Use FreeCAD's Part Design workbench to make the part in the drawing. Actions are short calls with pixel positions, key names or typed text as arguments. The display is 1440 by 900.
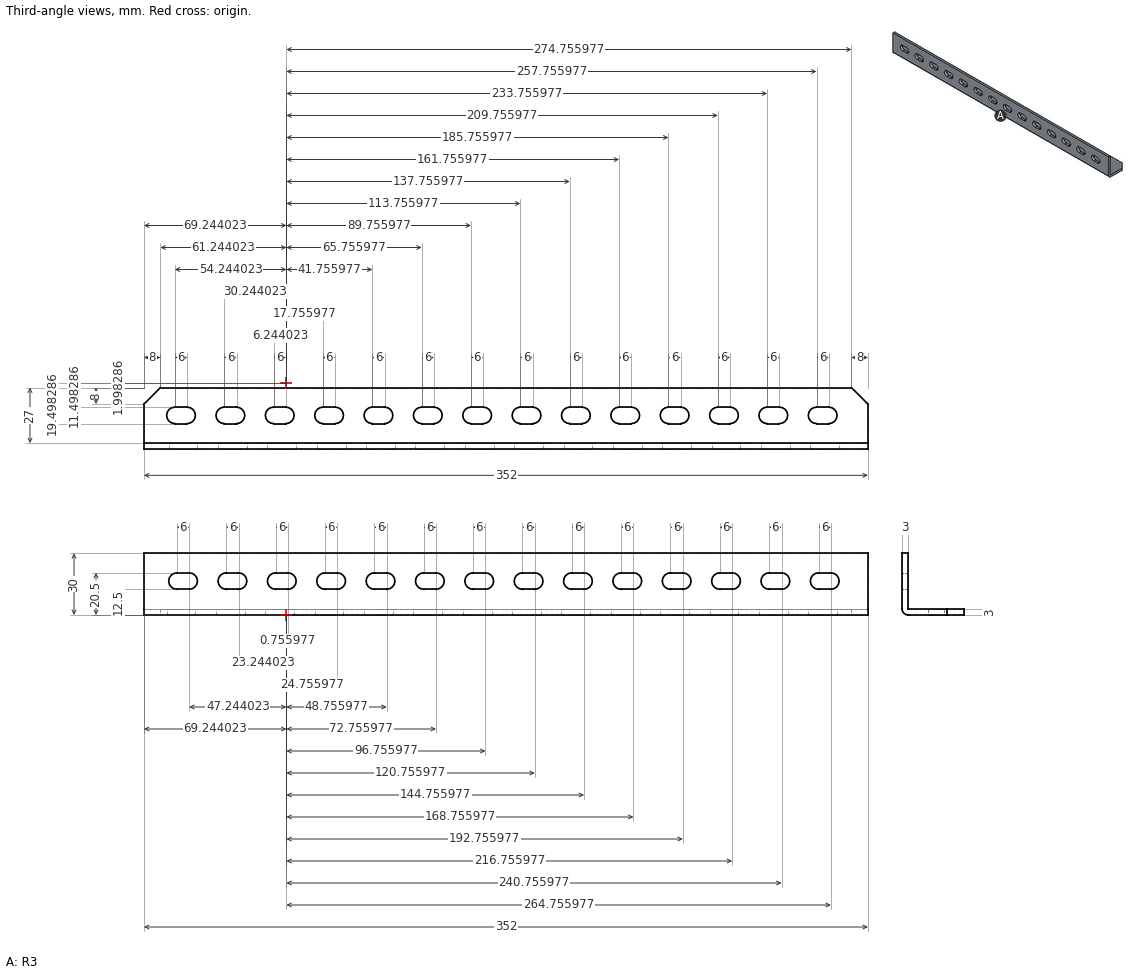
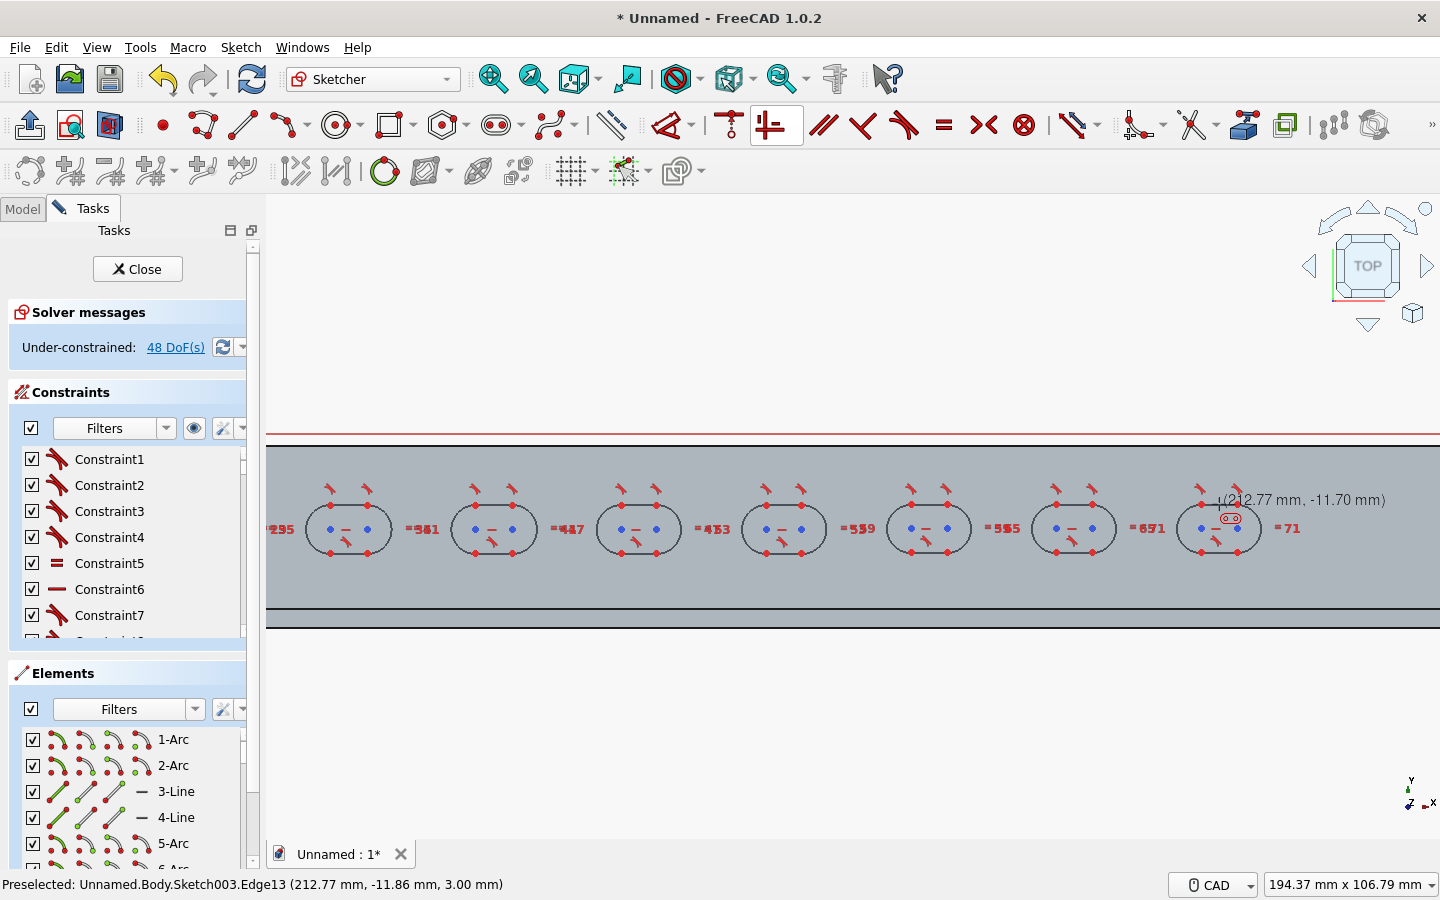
scroll(911, 530, down, 5)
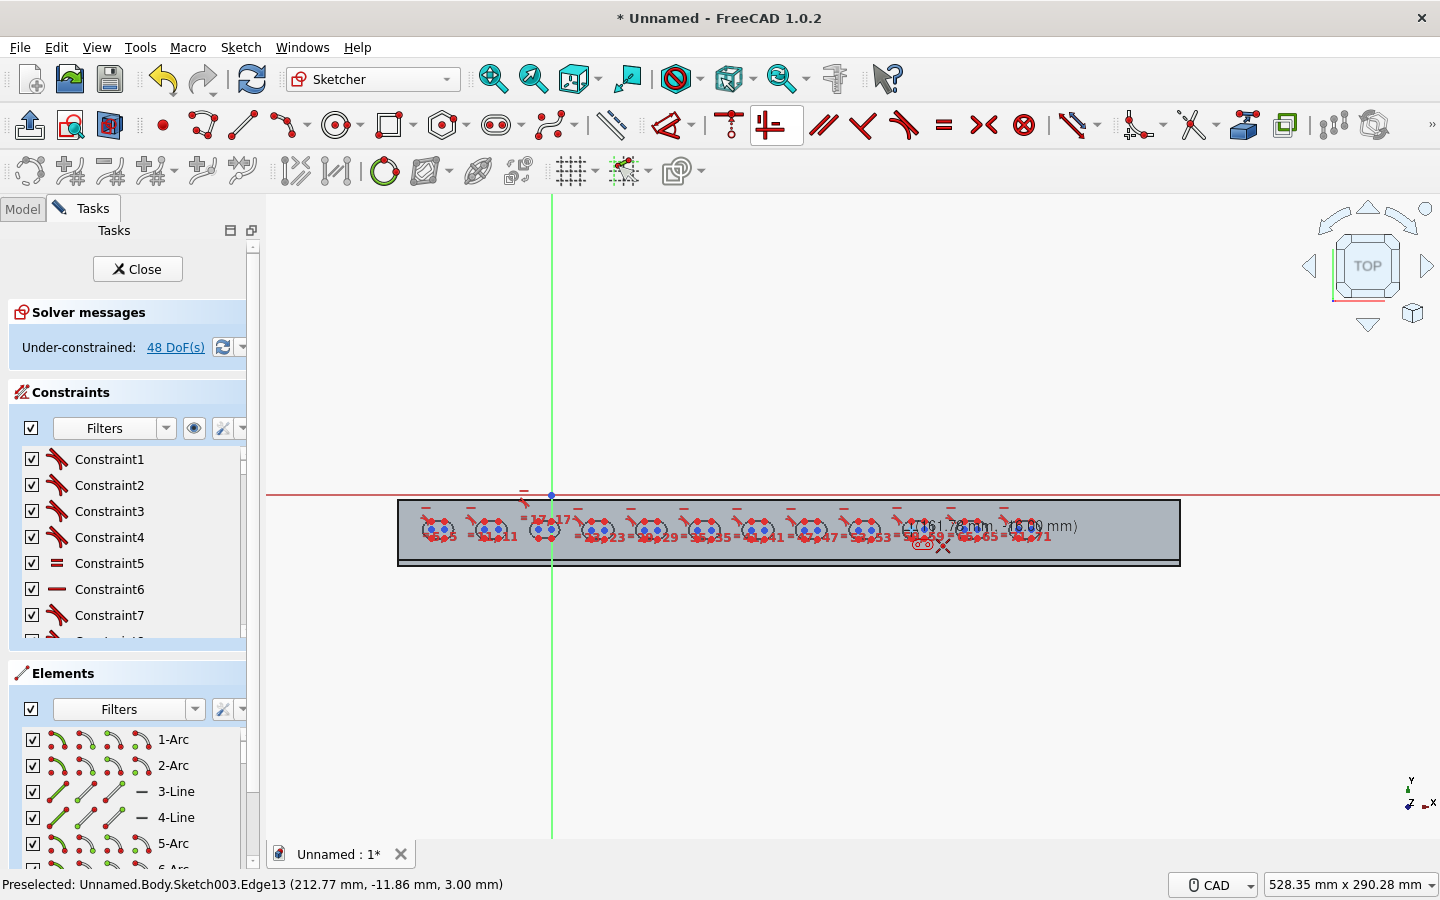
scroll(1071, 530, up, 5)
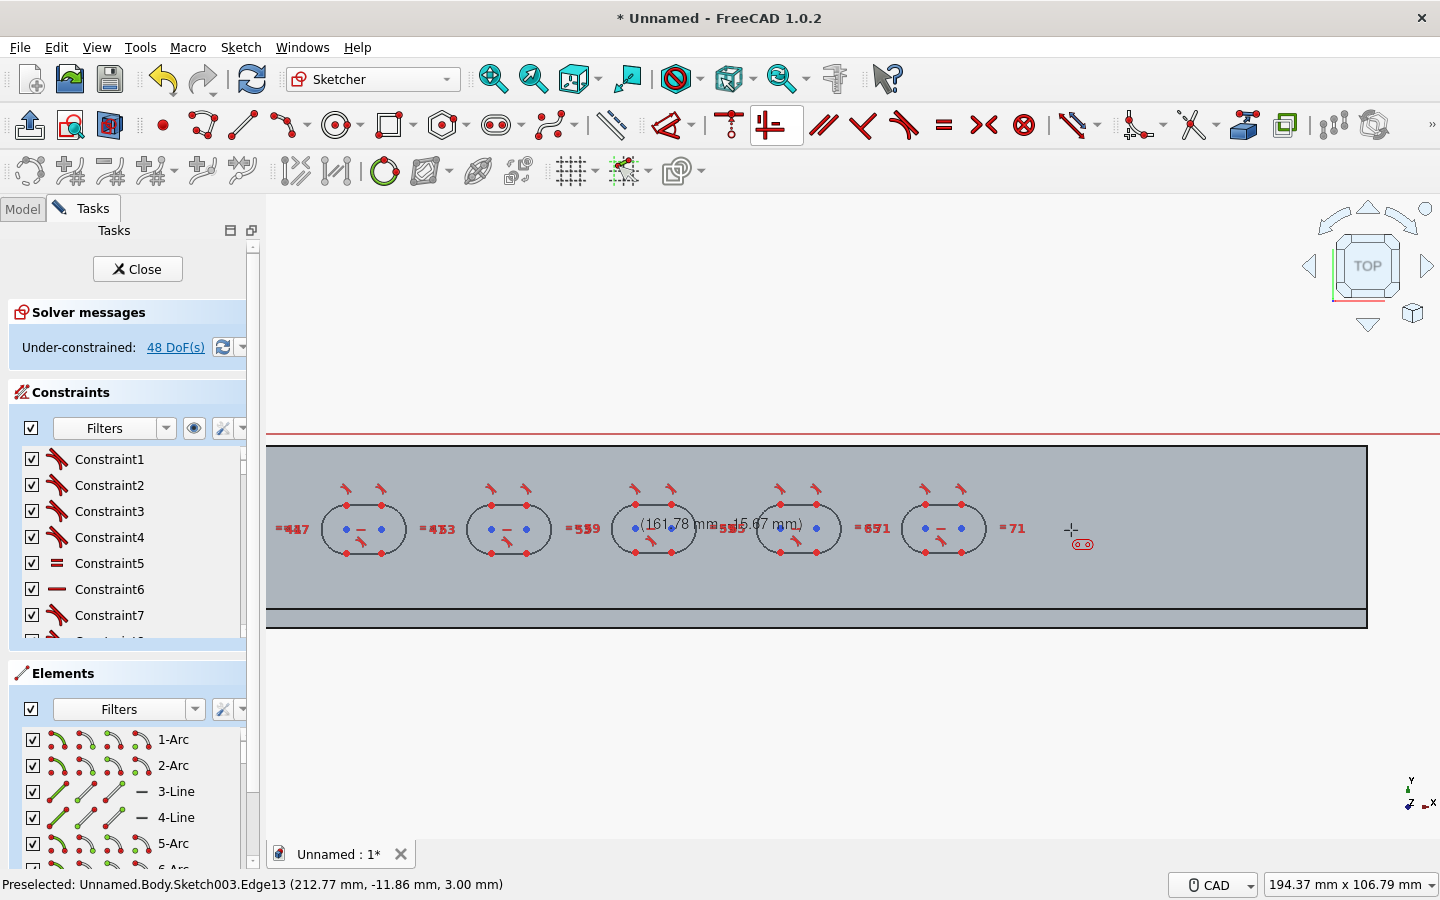
click(1071, 528)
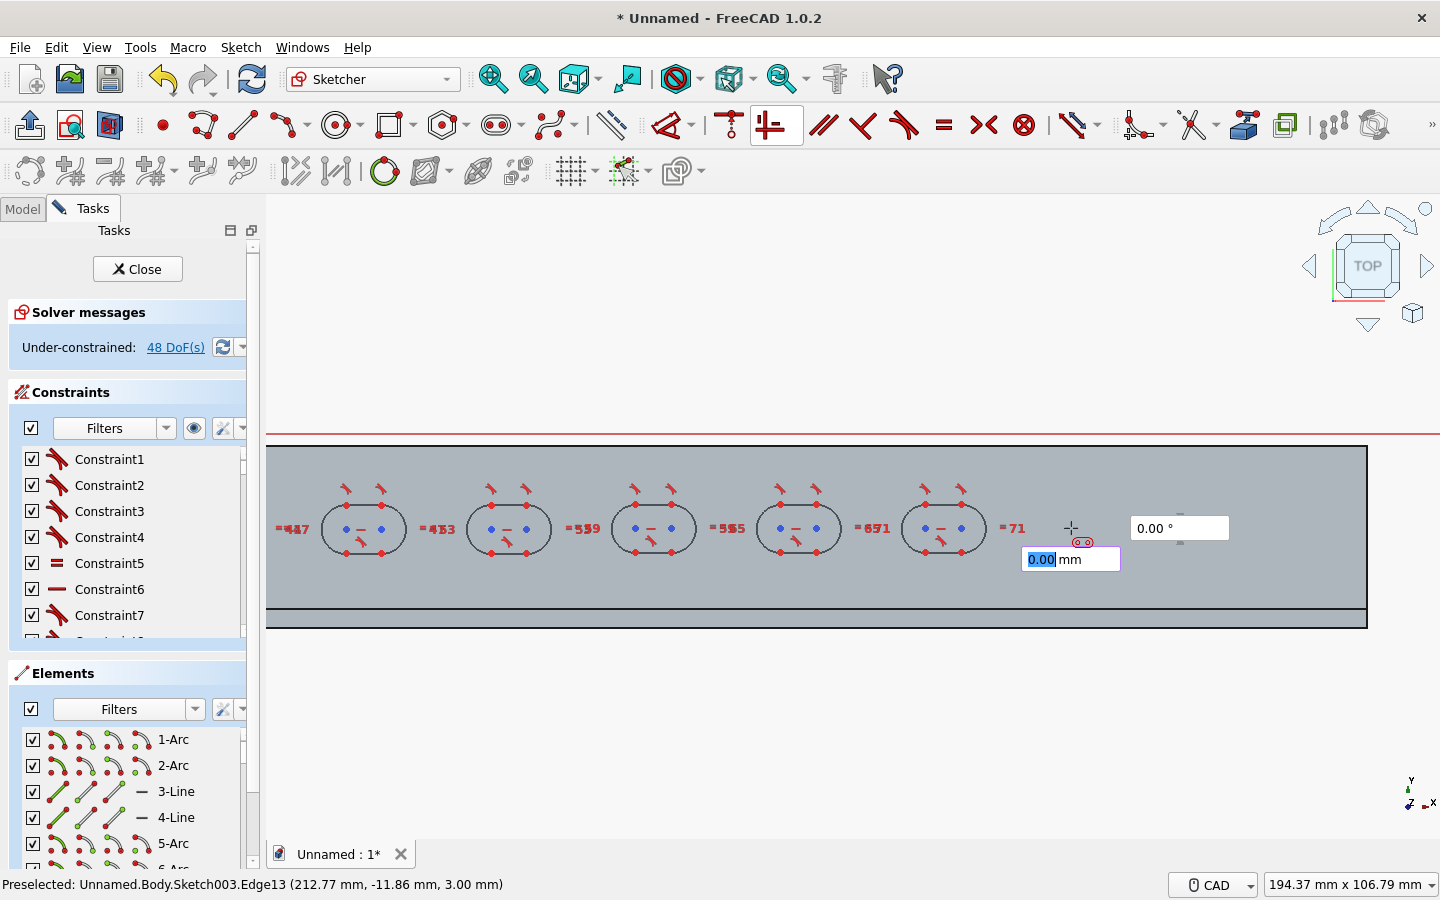
click(1107, 528)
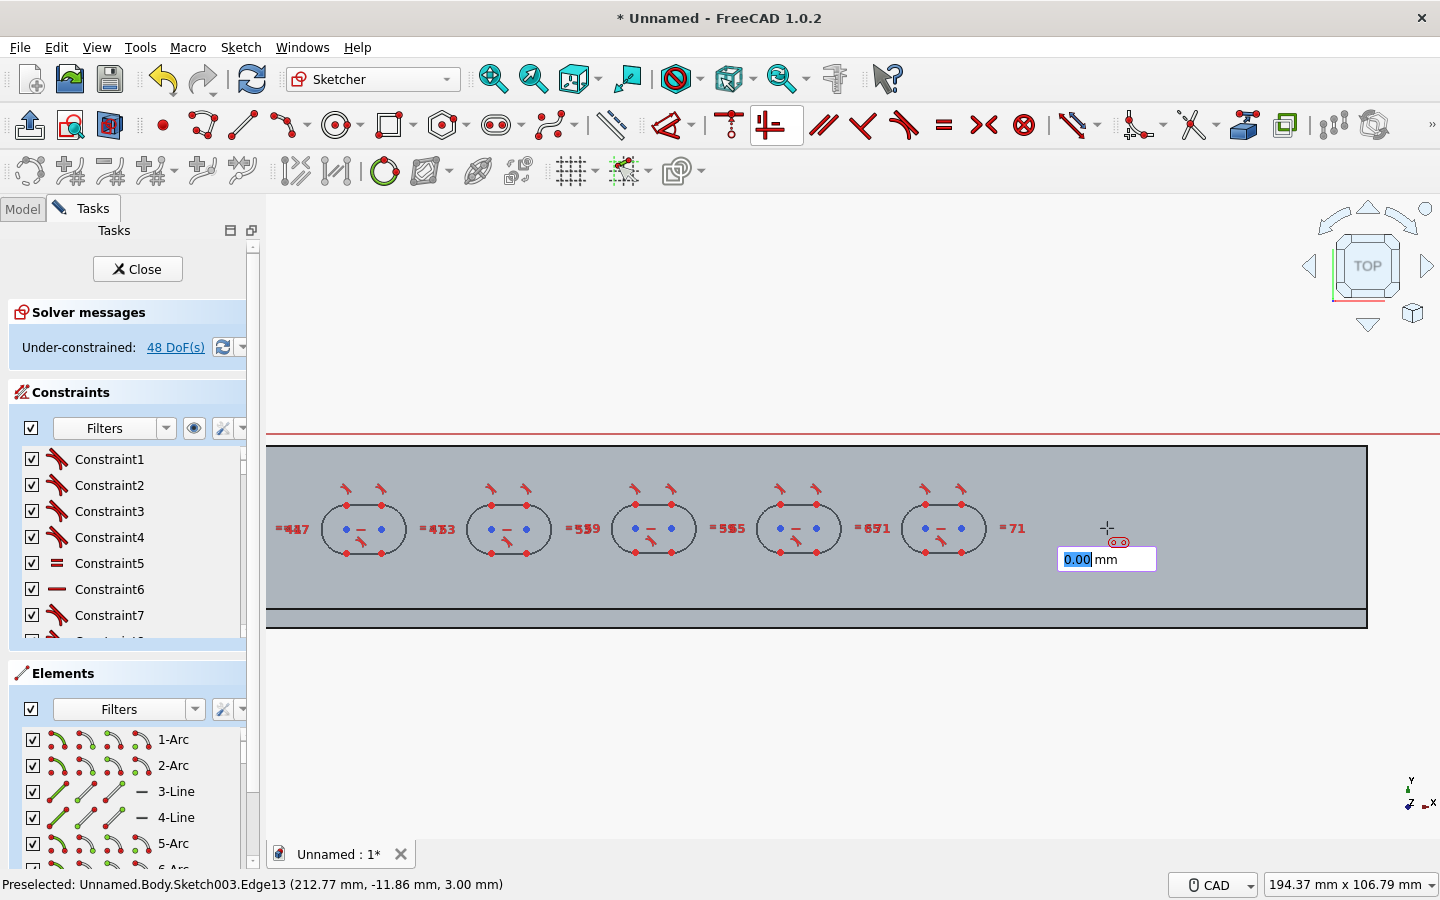
click(1089, 504)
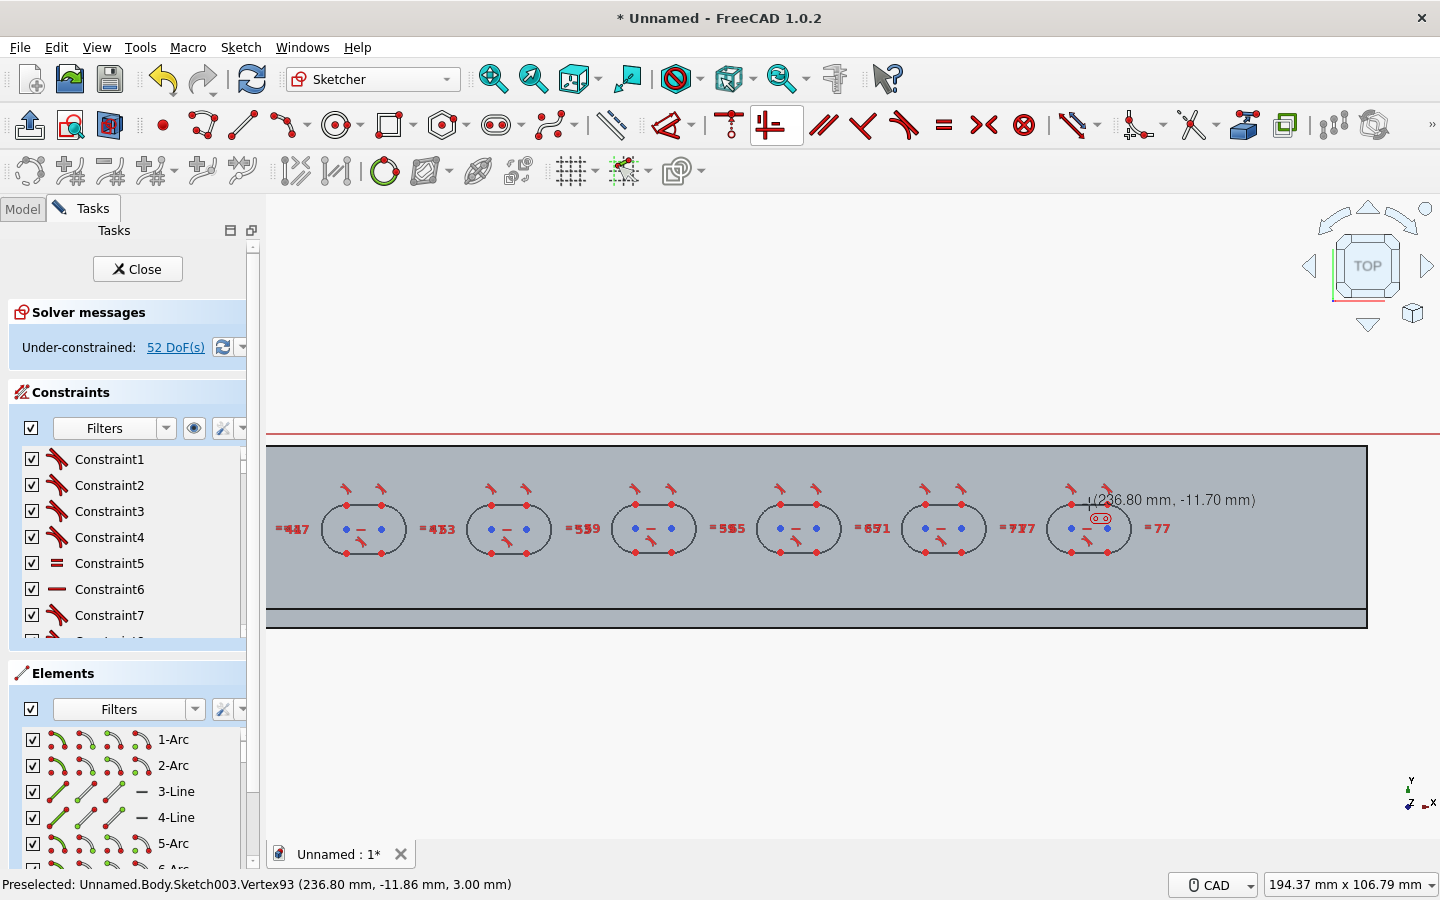
click(1216, 528)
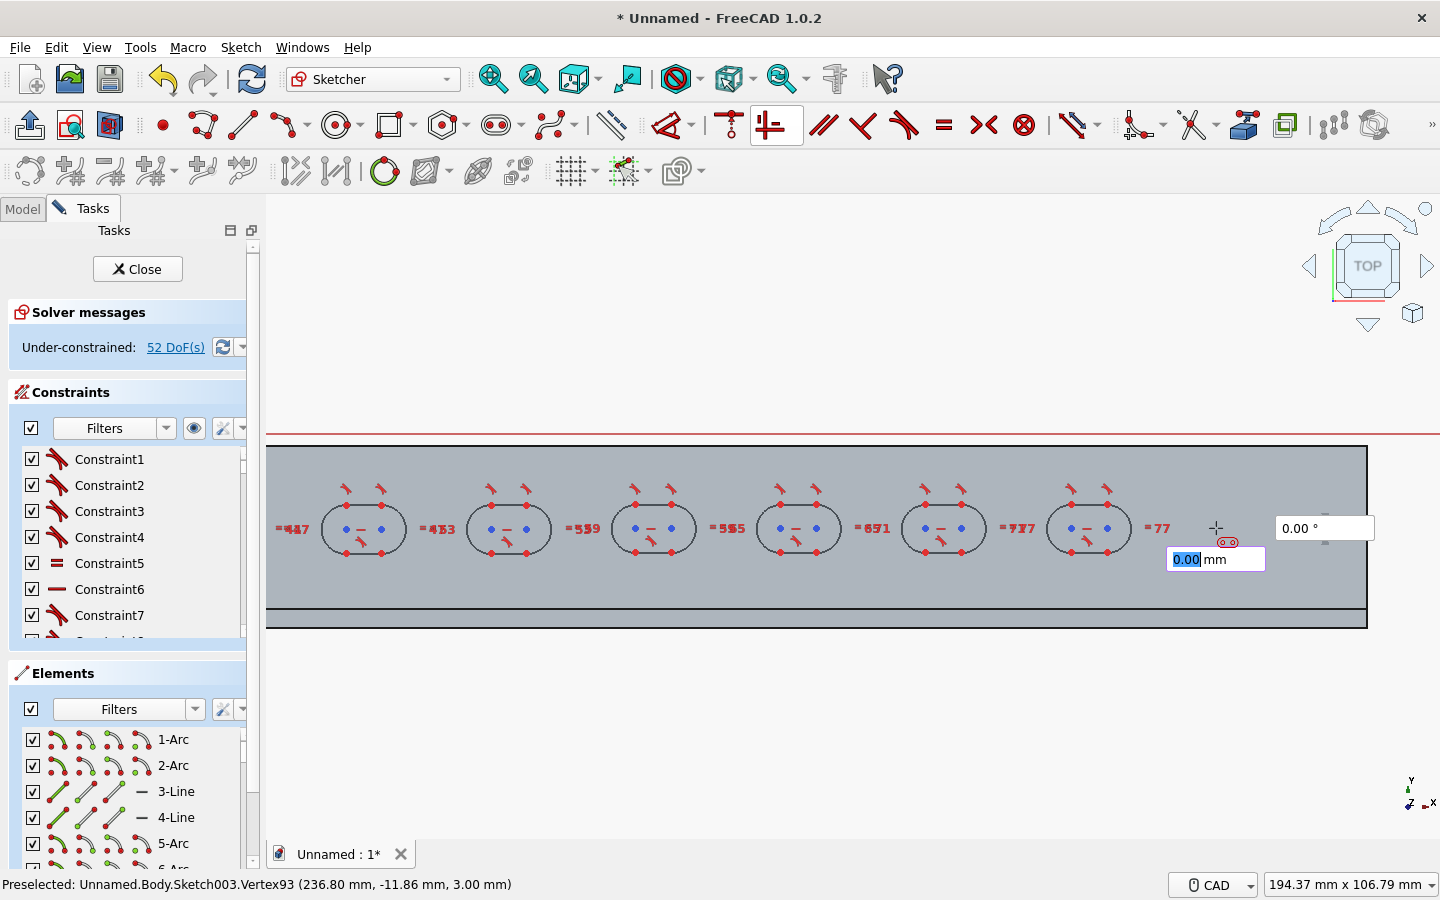
click(1252, 528)